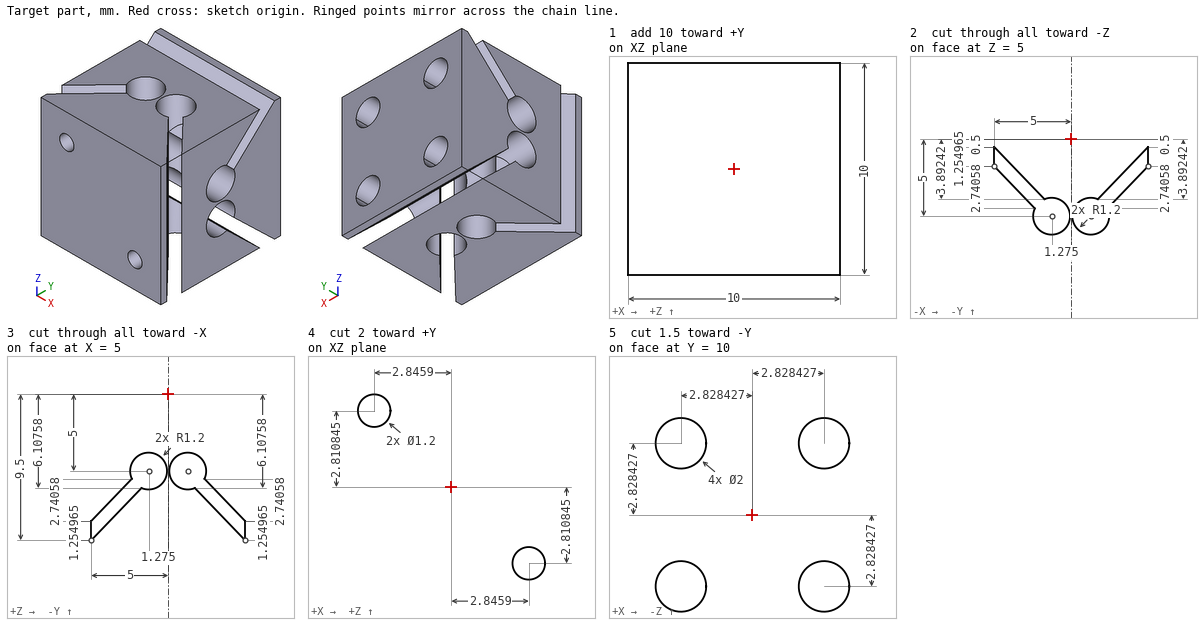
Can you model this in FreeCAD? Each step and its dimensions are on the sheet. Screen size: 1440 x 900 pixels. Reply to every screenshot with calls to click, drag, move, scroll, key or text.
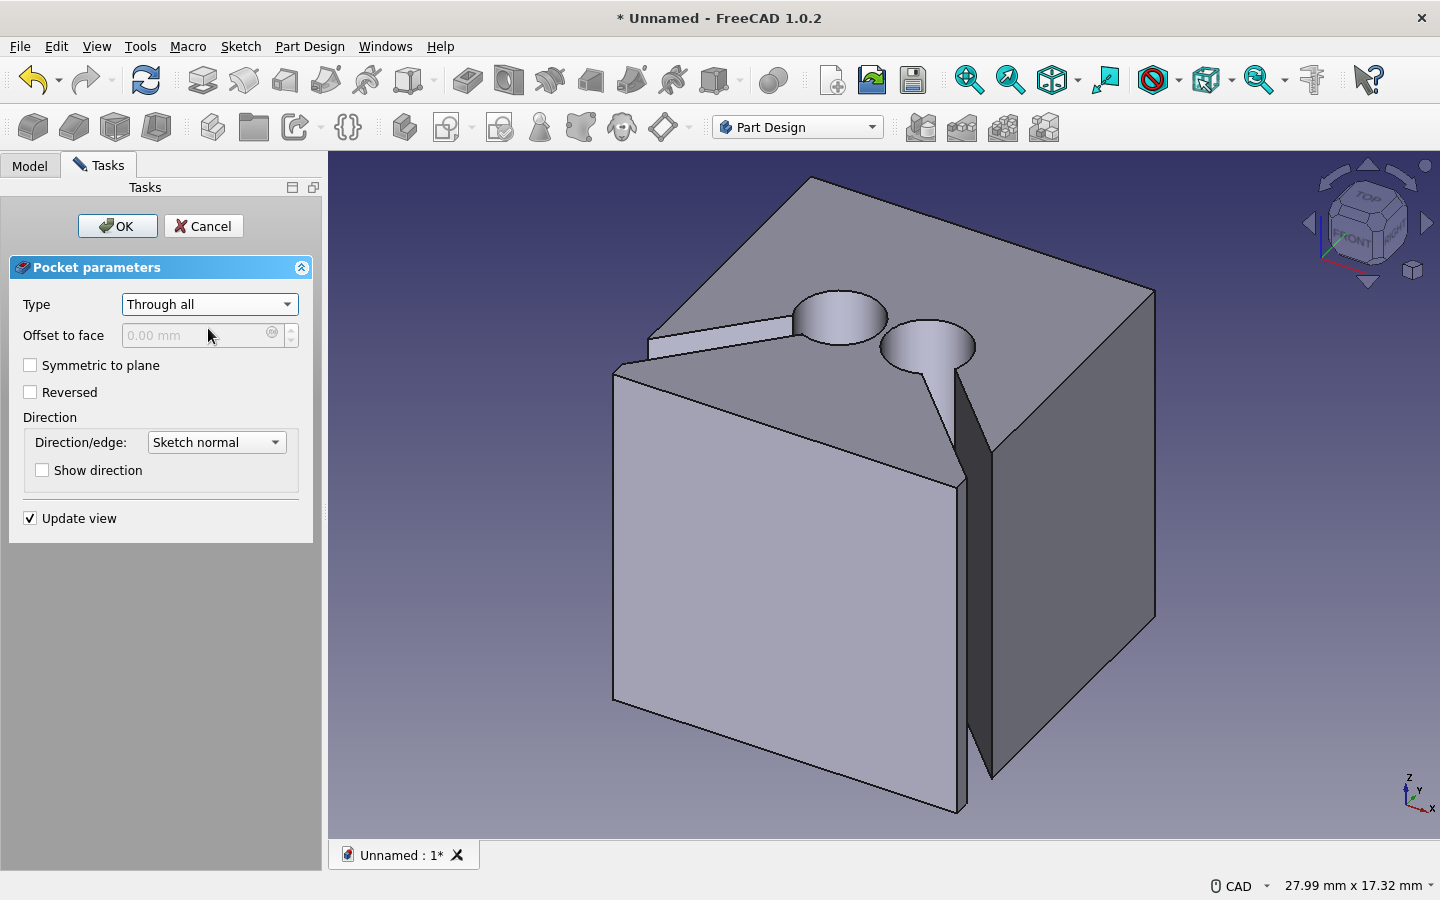
click(118, 226)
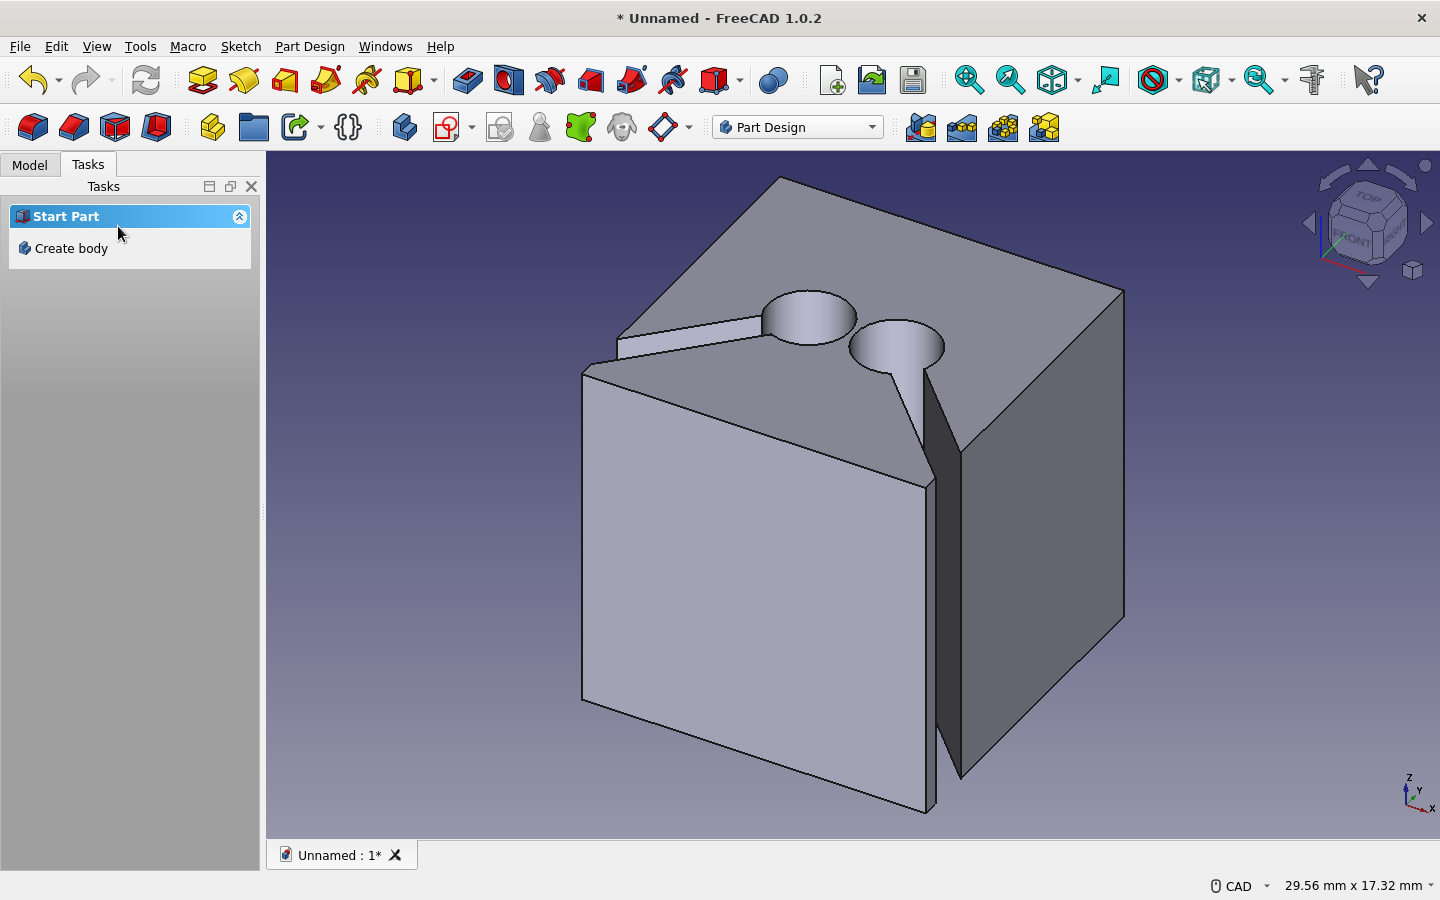
click(1042, 534)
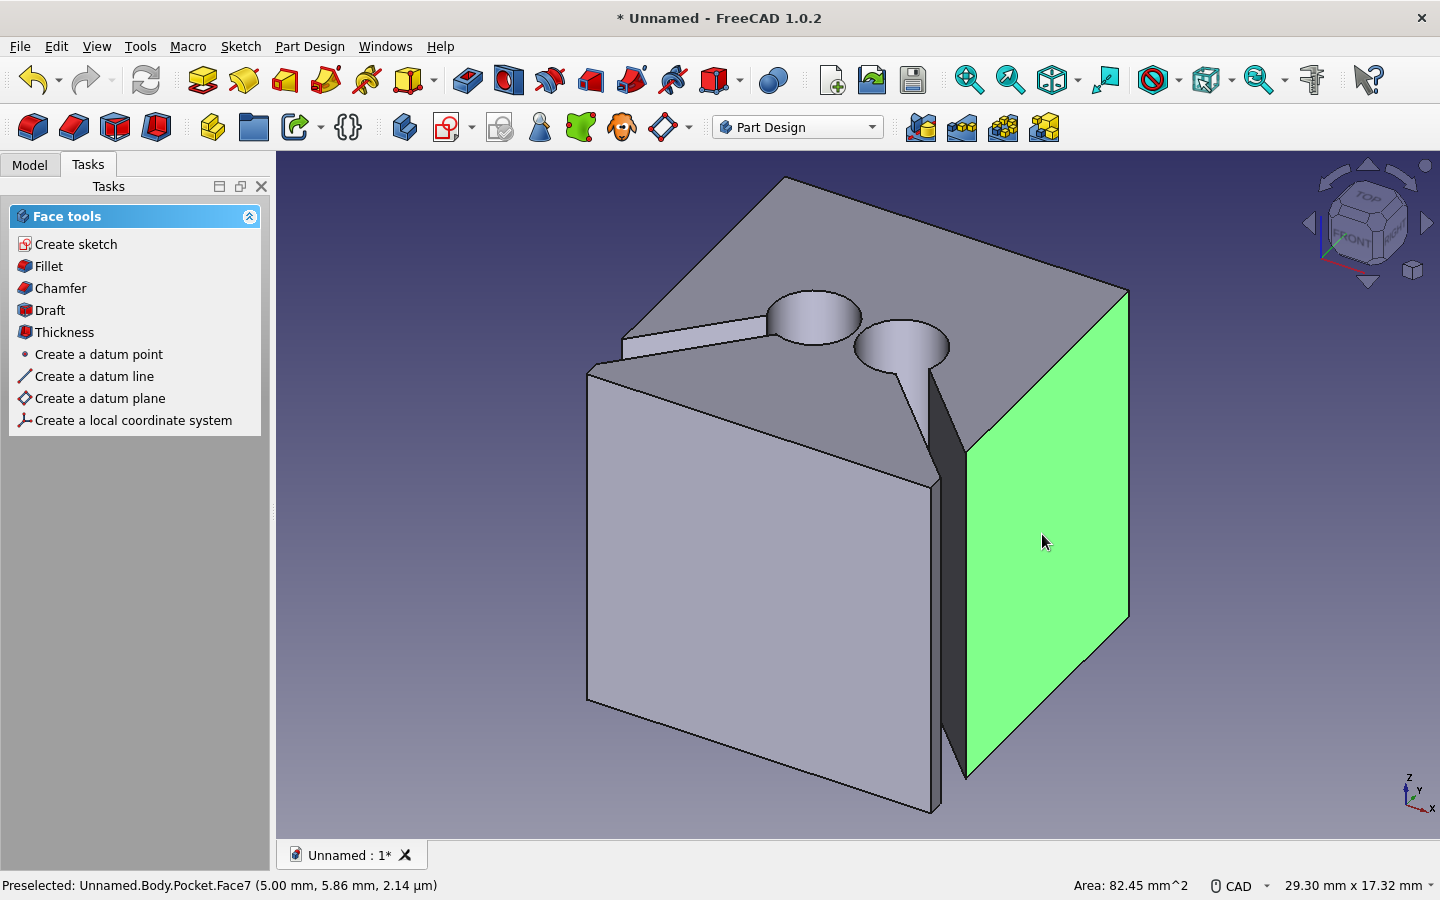
click(446, 128)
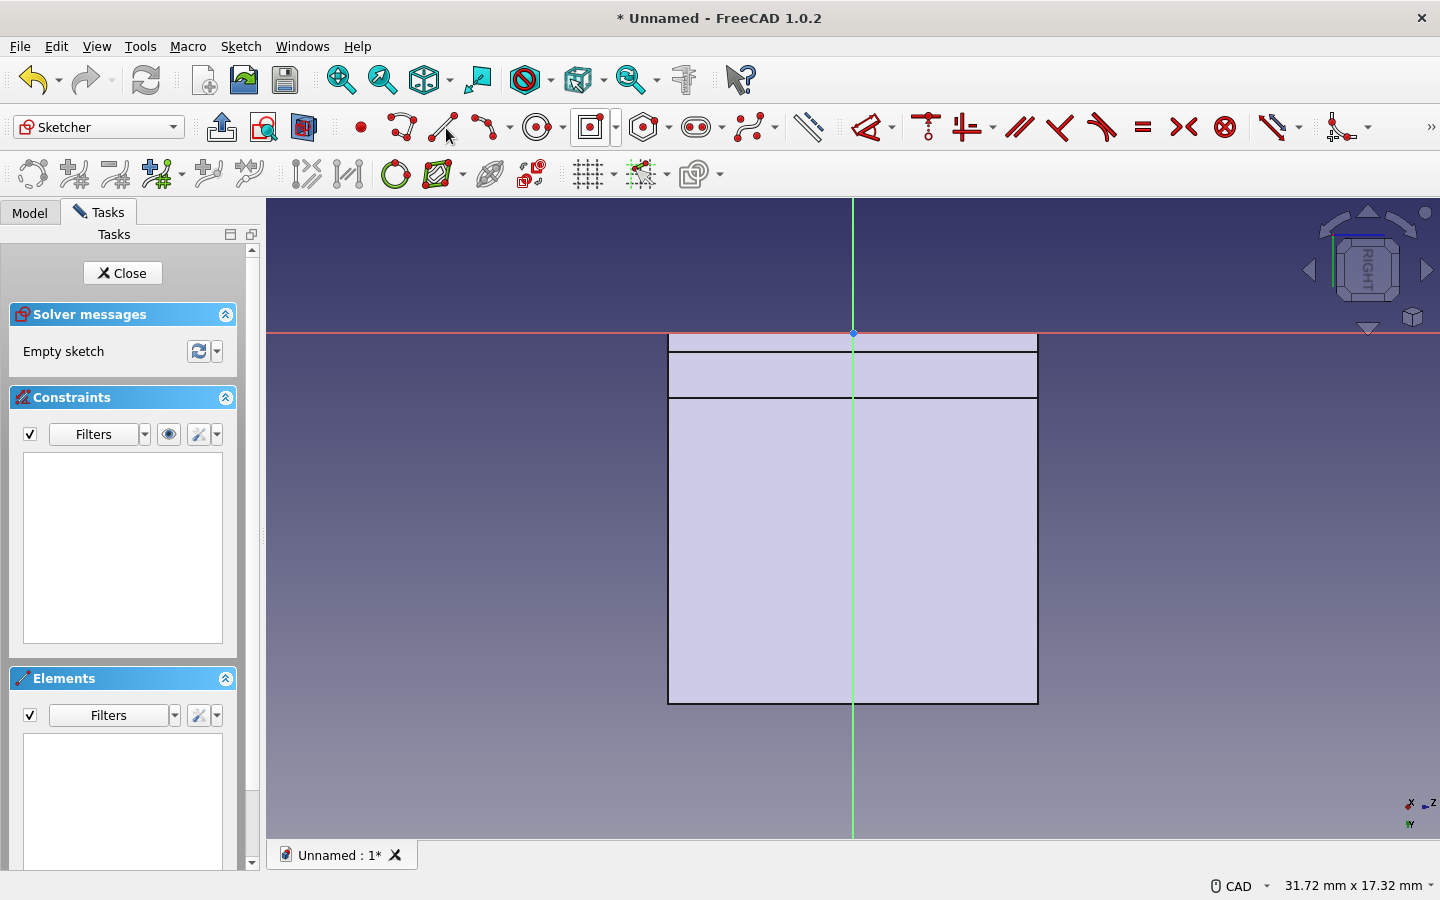
click(402, 128)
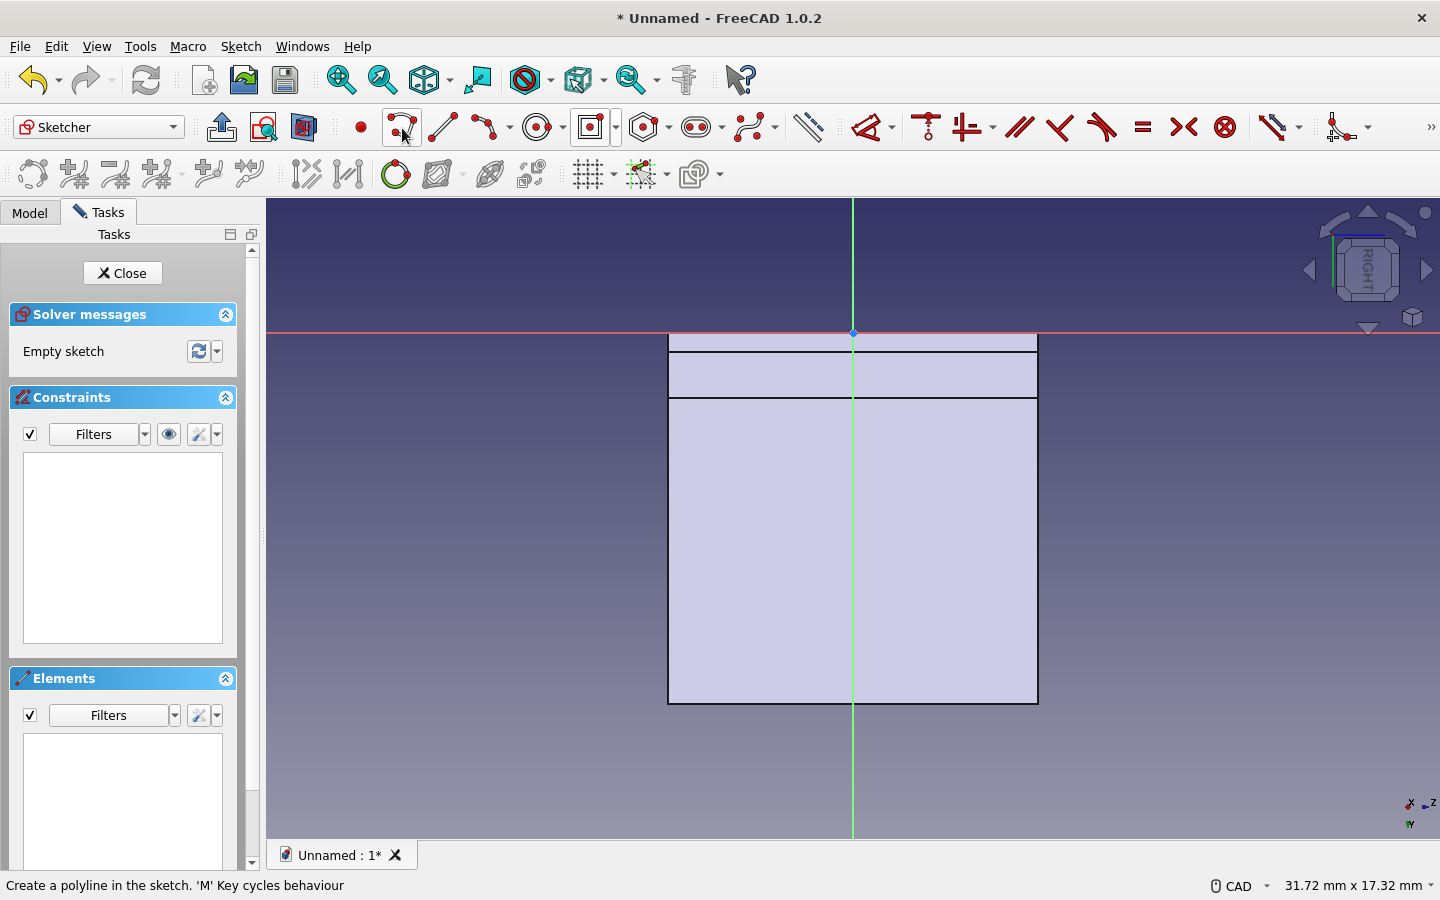
click(766, 537)
click(668, 639)
click(668, 685)
click(789, 559)
right_click(789, 559)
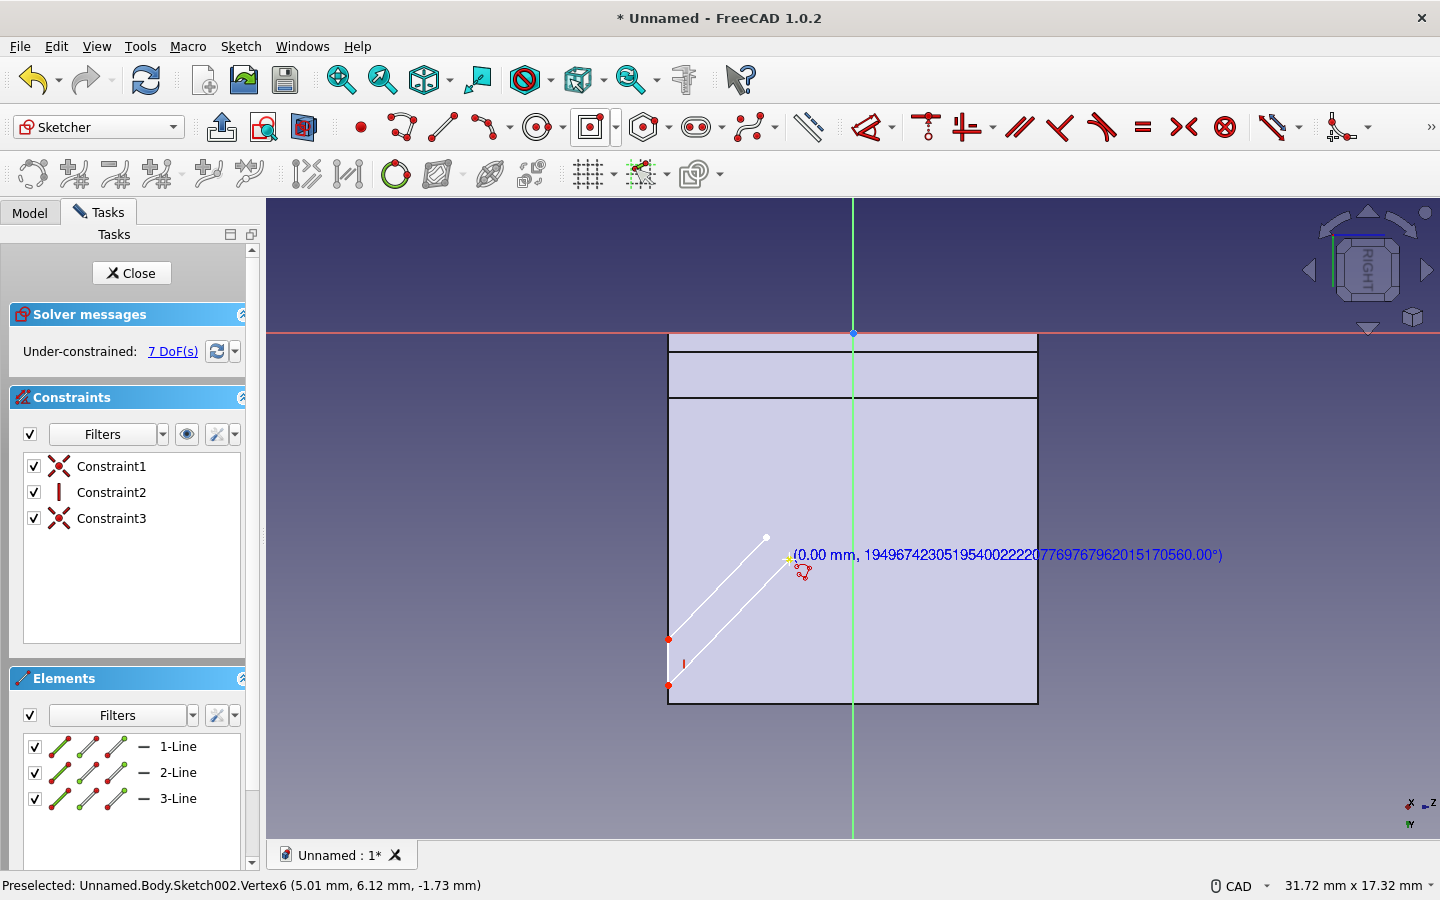
key(g)
key(3)
key(a)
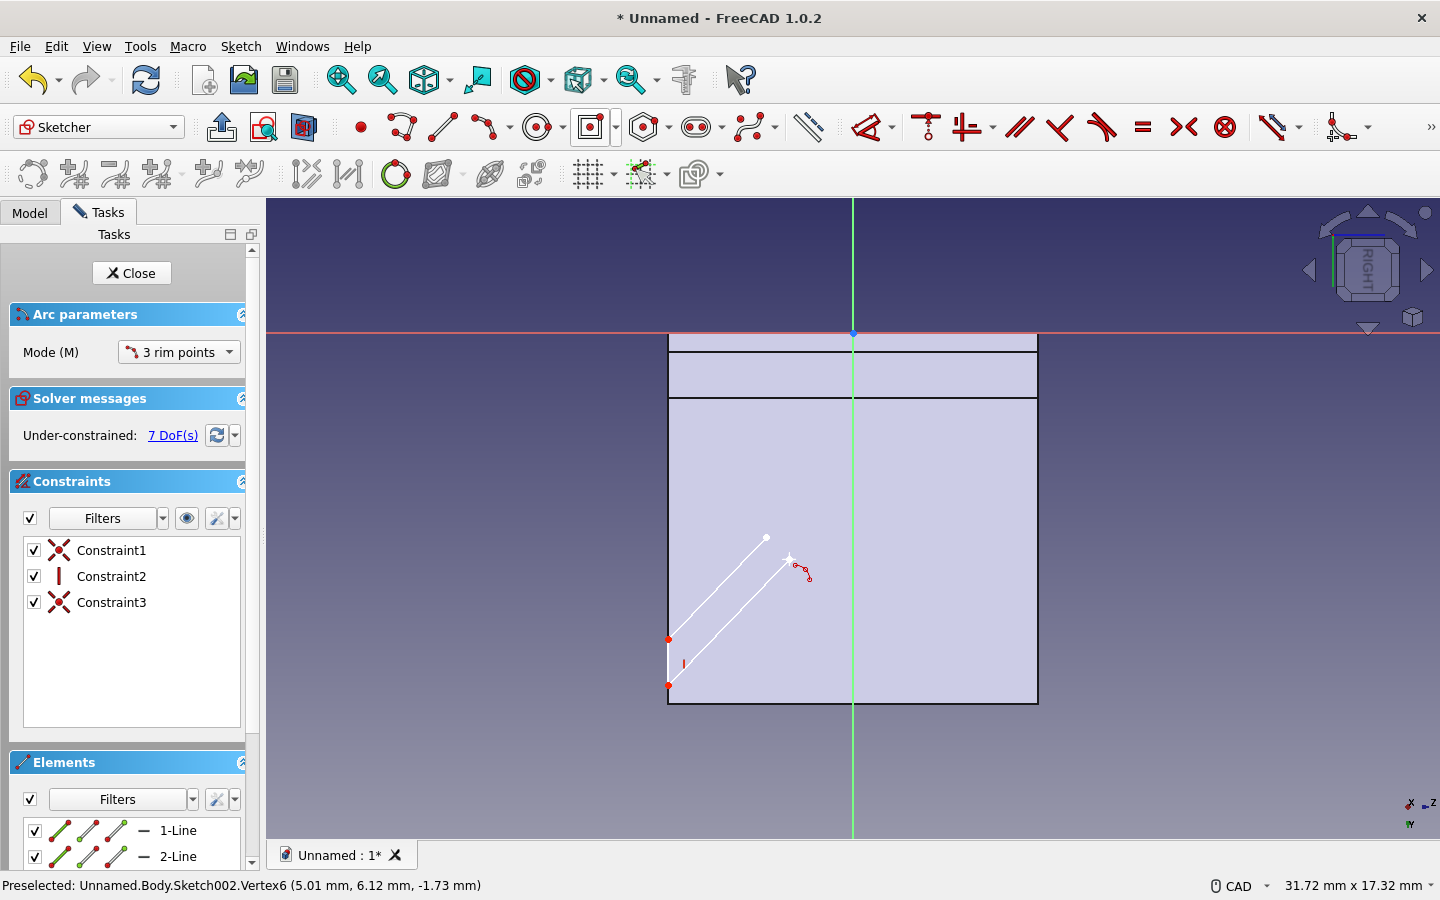
click(789, 560)
click(766, 538)
click(837, 486)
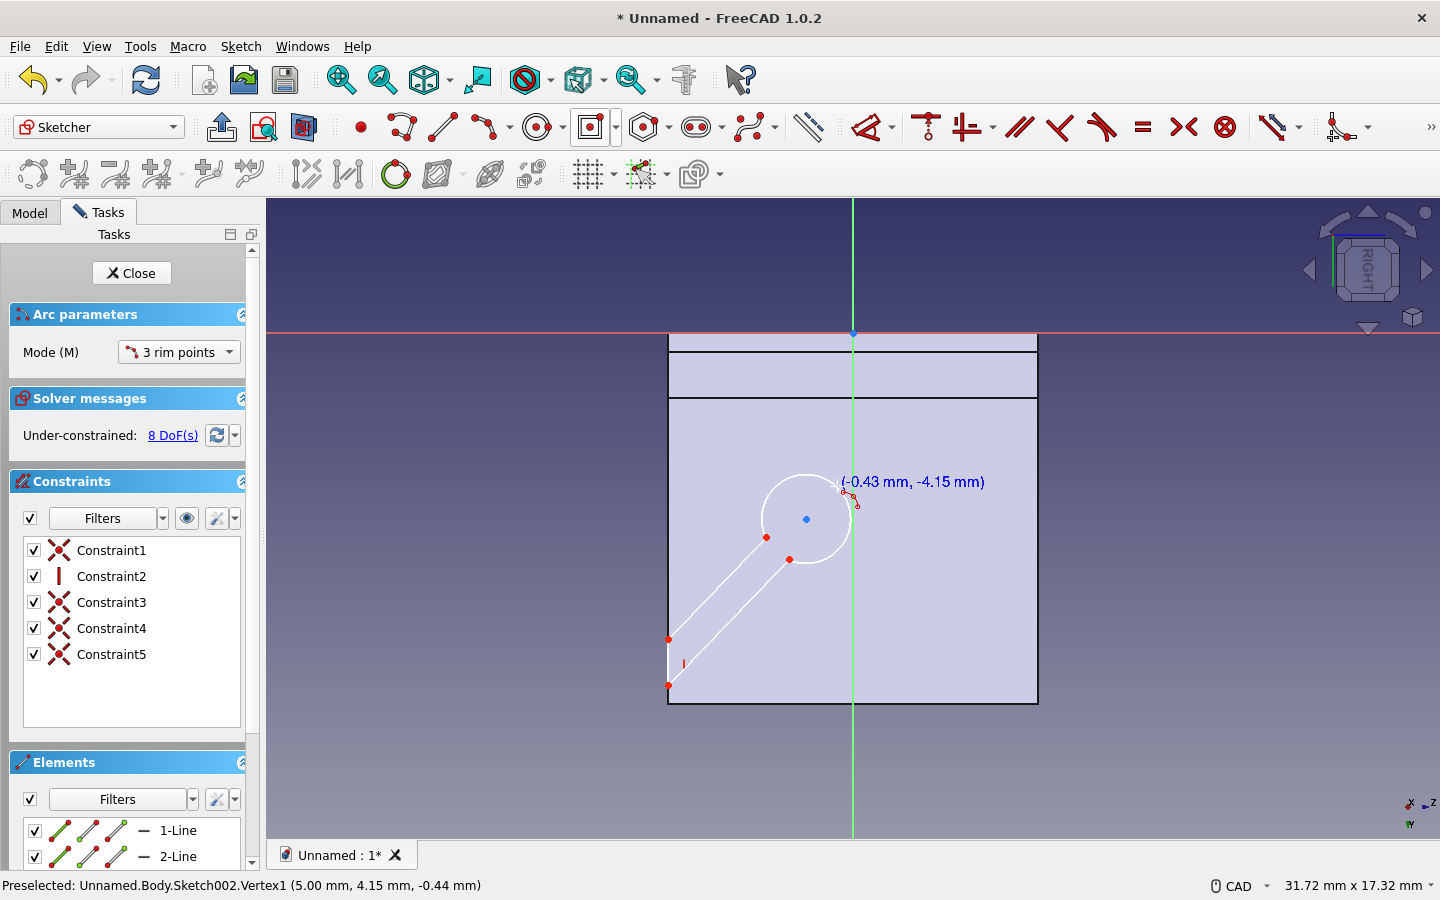
click(402, 128)